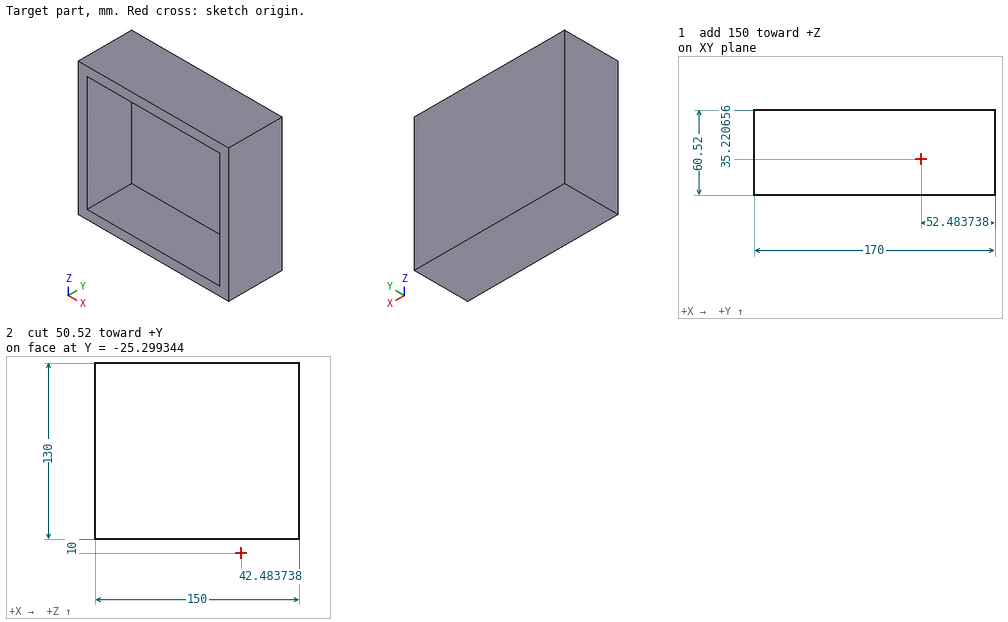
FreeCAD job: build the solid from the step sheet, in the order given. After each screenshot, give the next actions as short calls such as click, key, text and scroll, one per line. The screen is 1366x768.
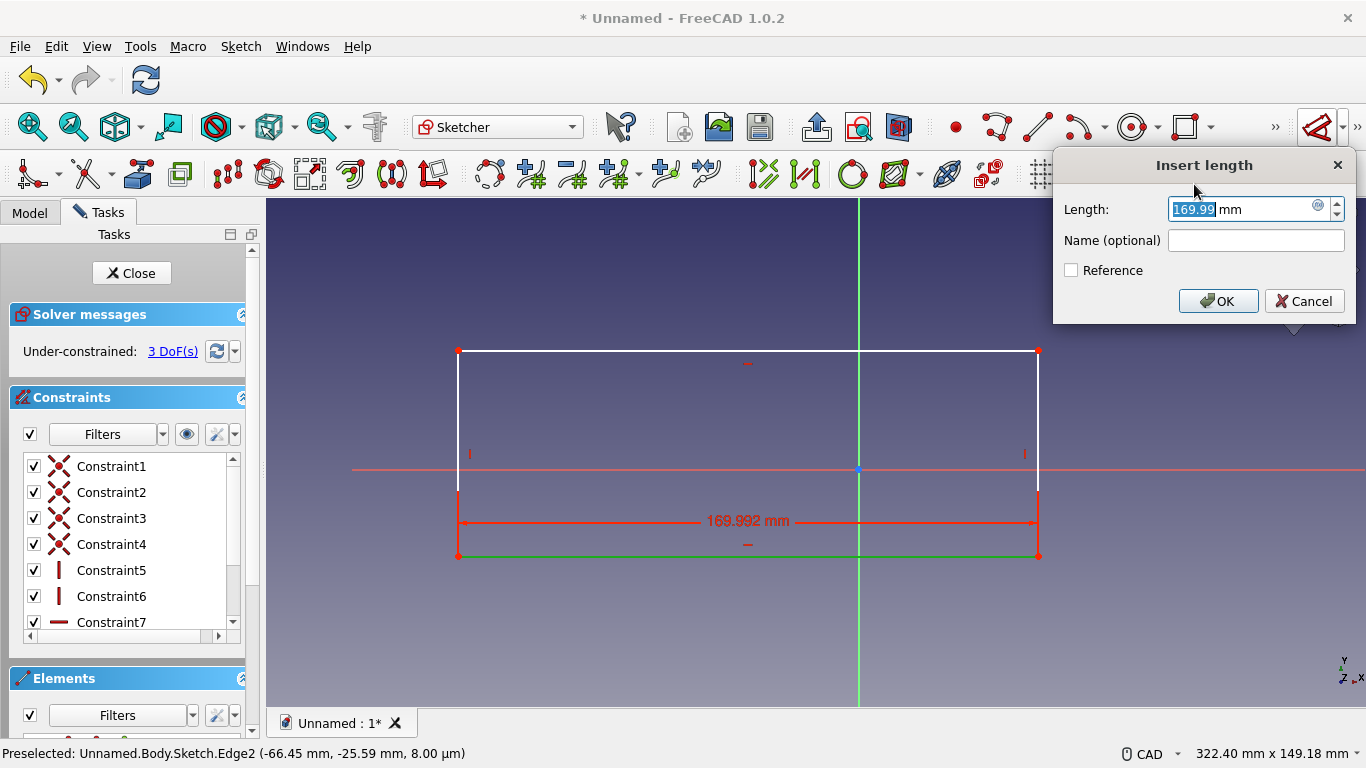
text(170)
key(Return)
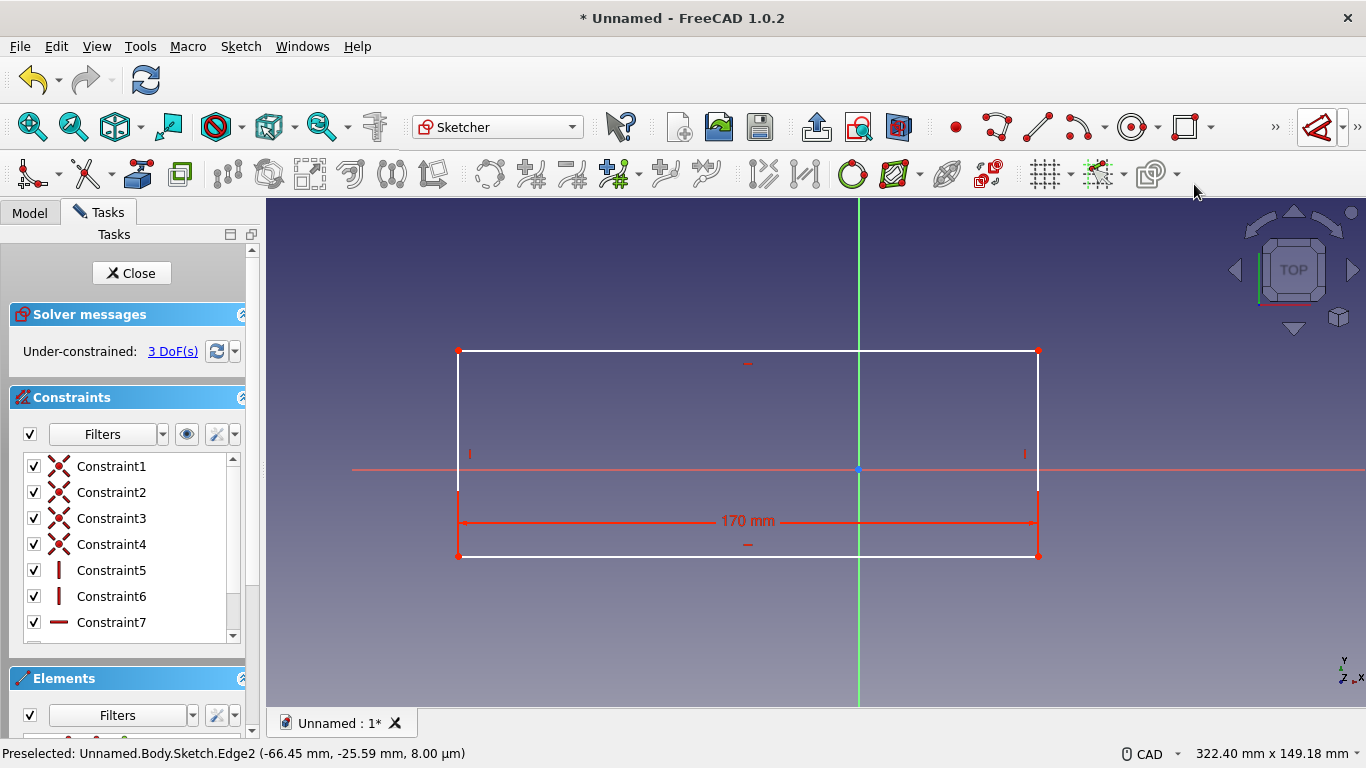
click(458, 413)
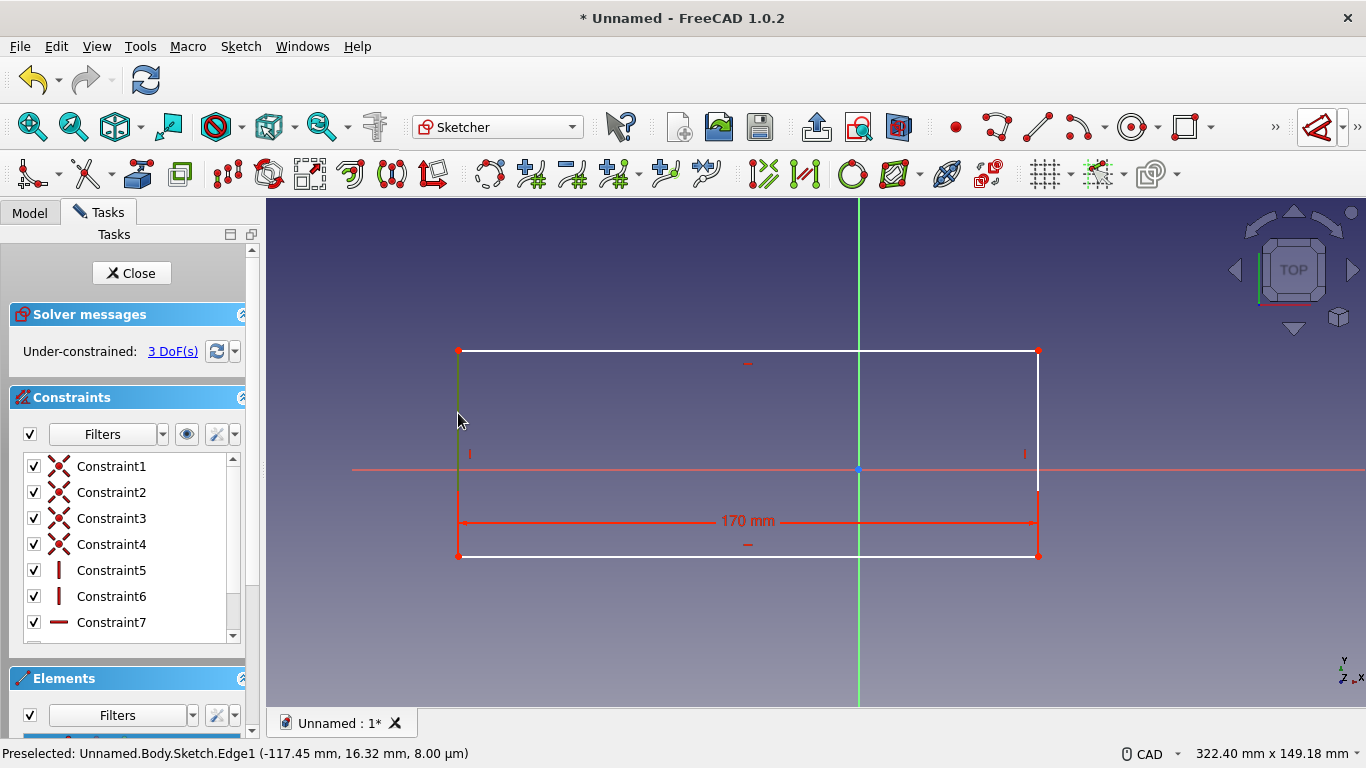
key(i)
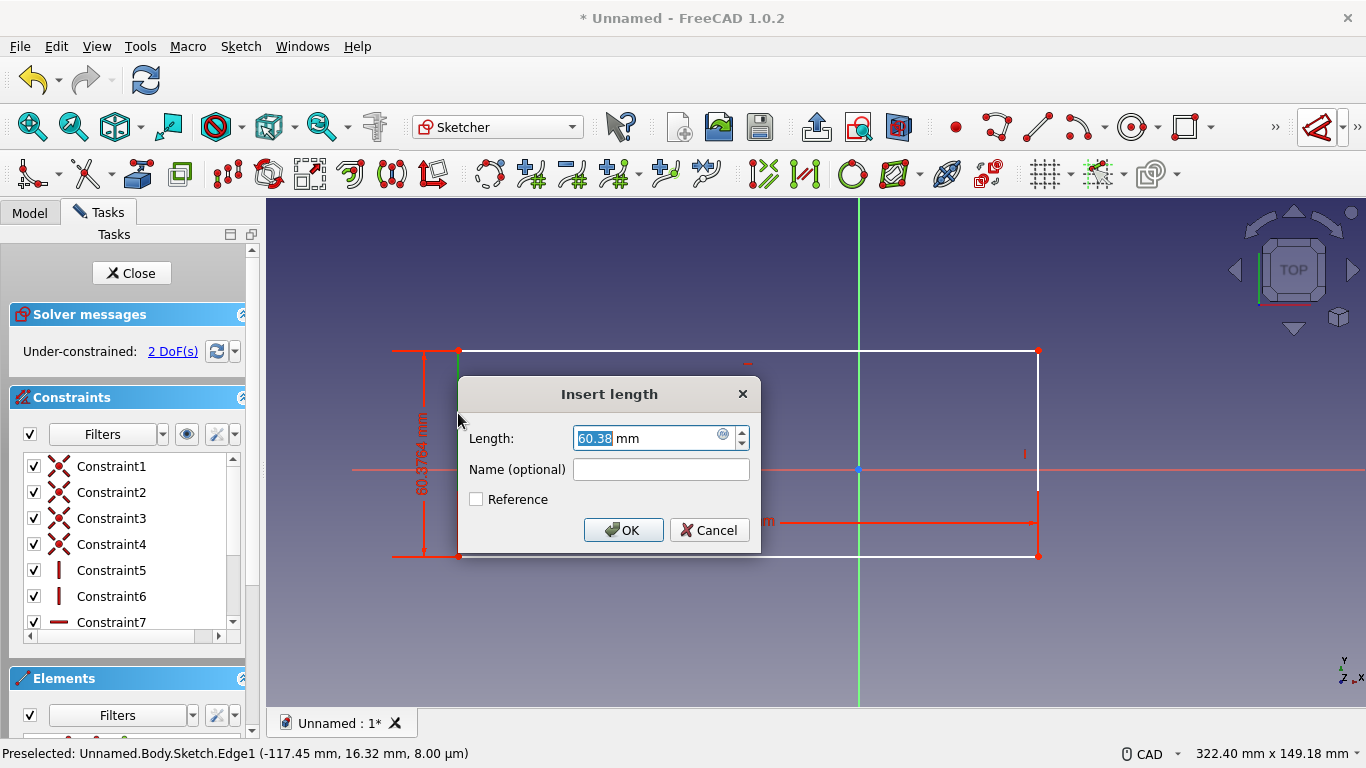
text(60.52)
key(Return)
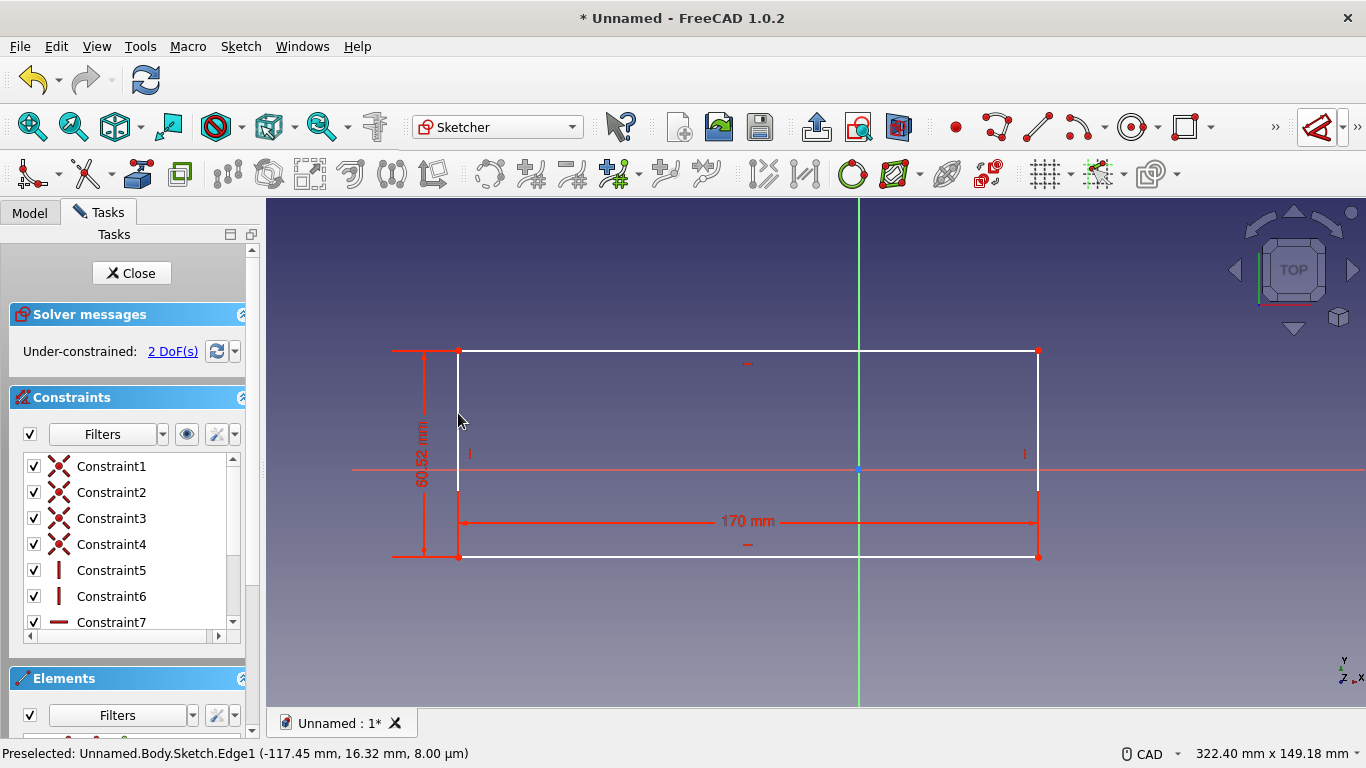
click(458, 351)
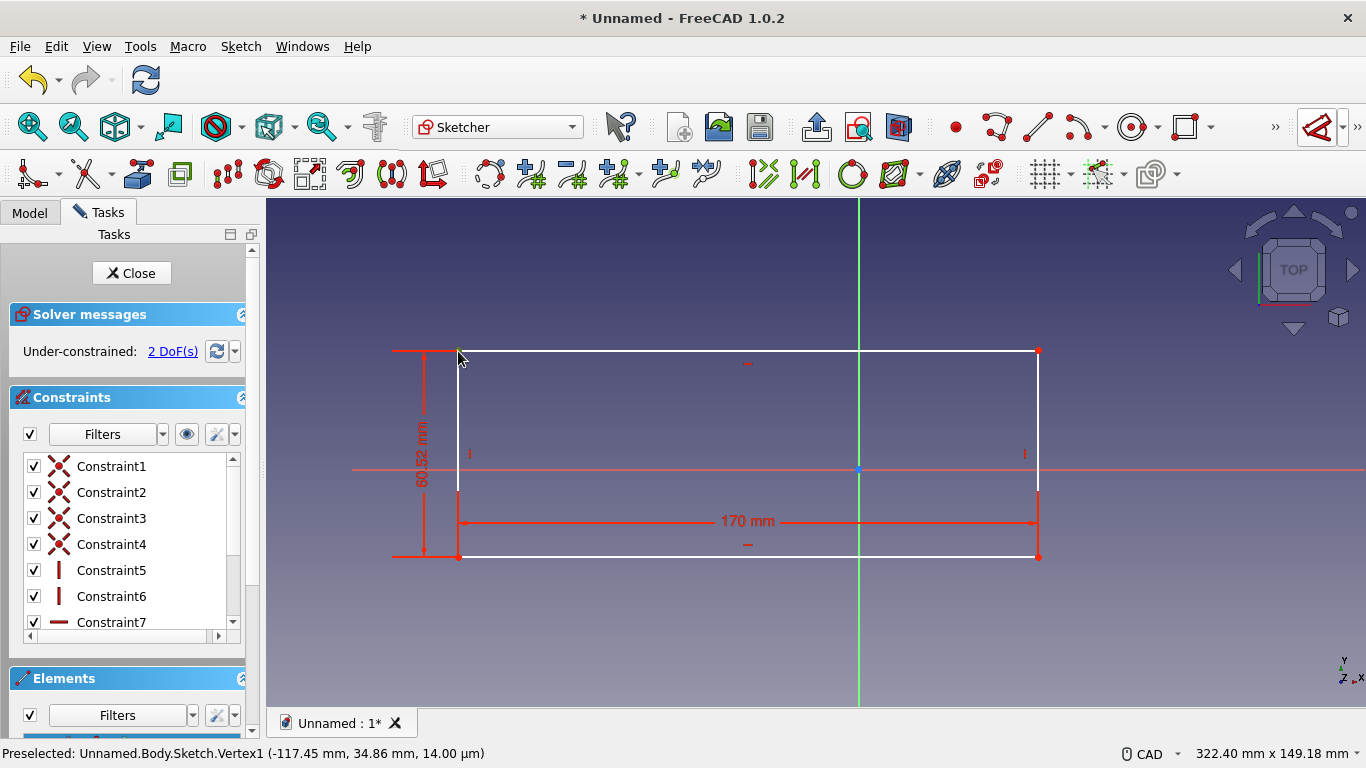
key(i)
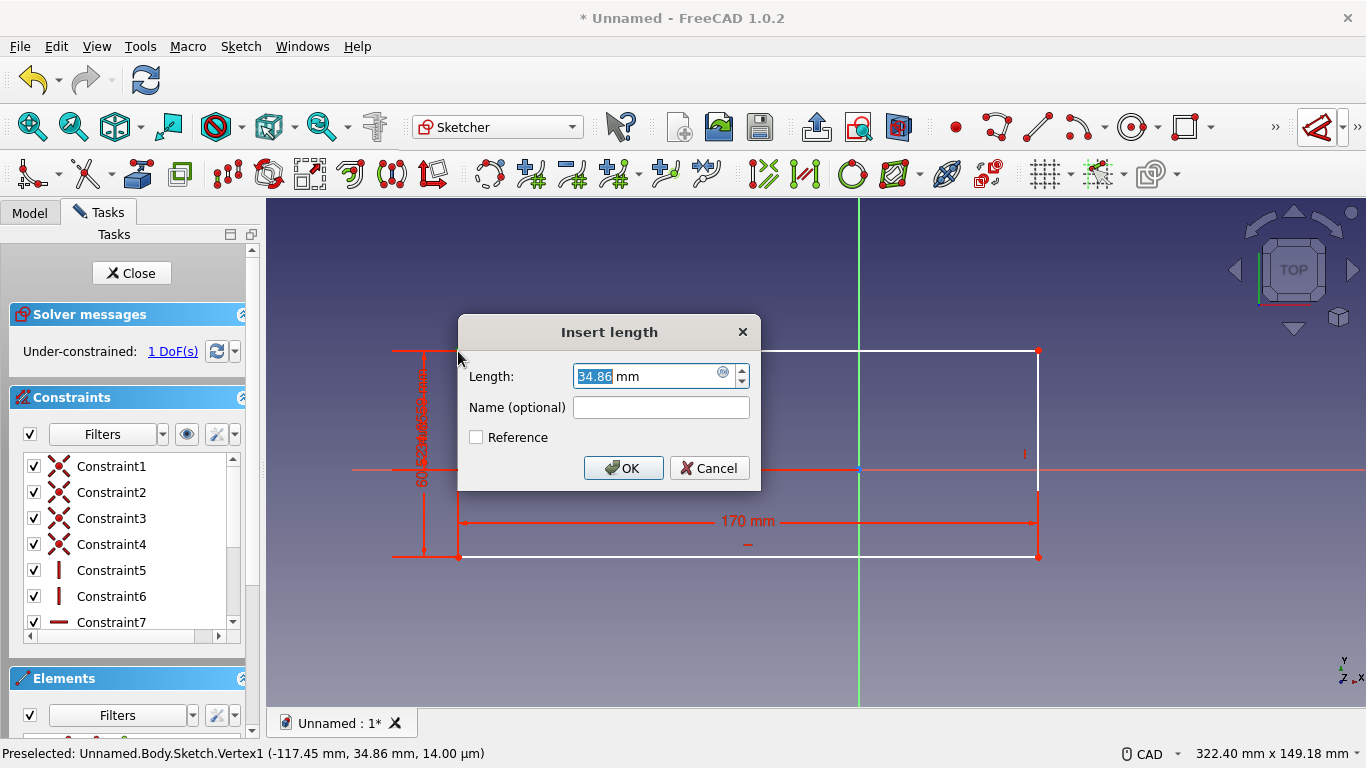
text(35.220656)
key(Return)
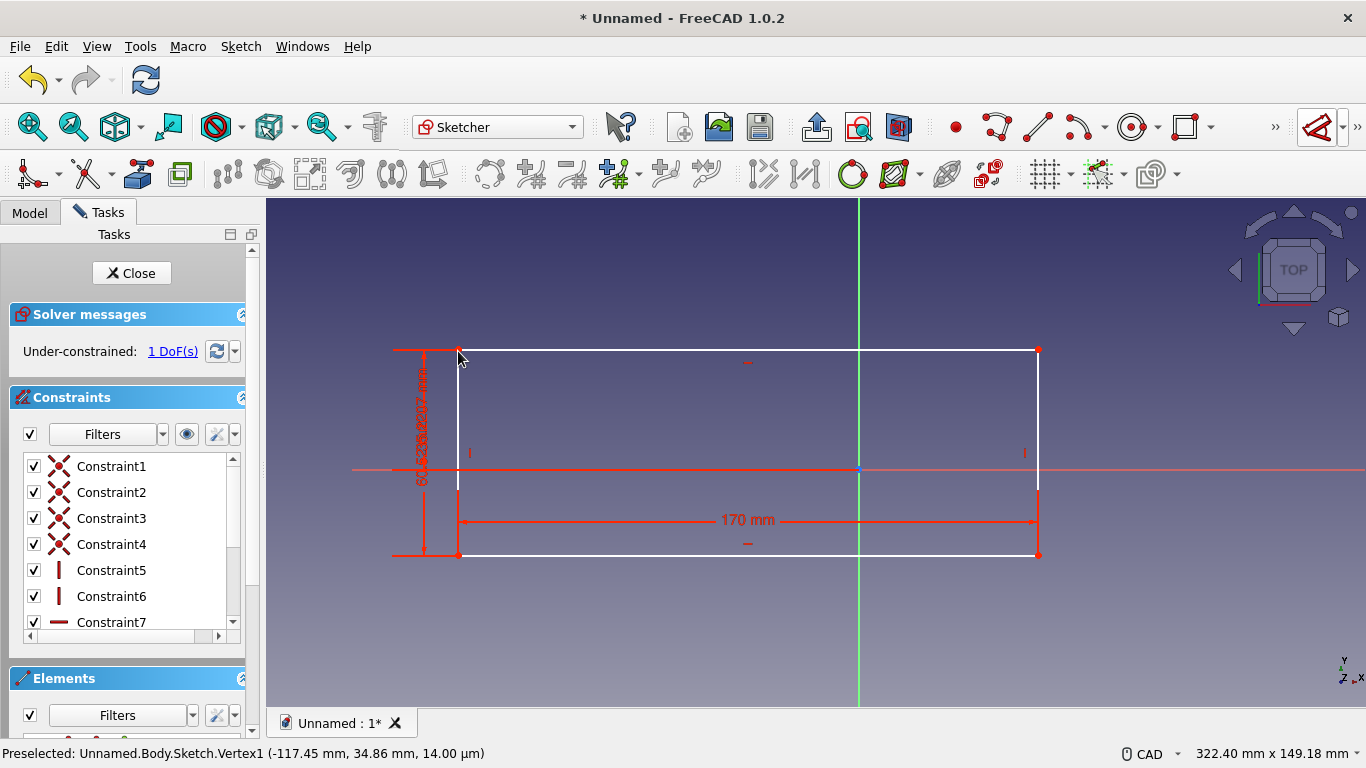
click(1038, 556)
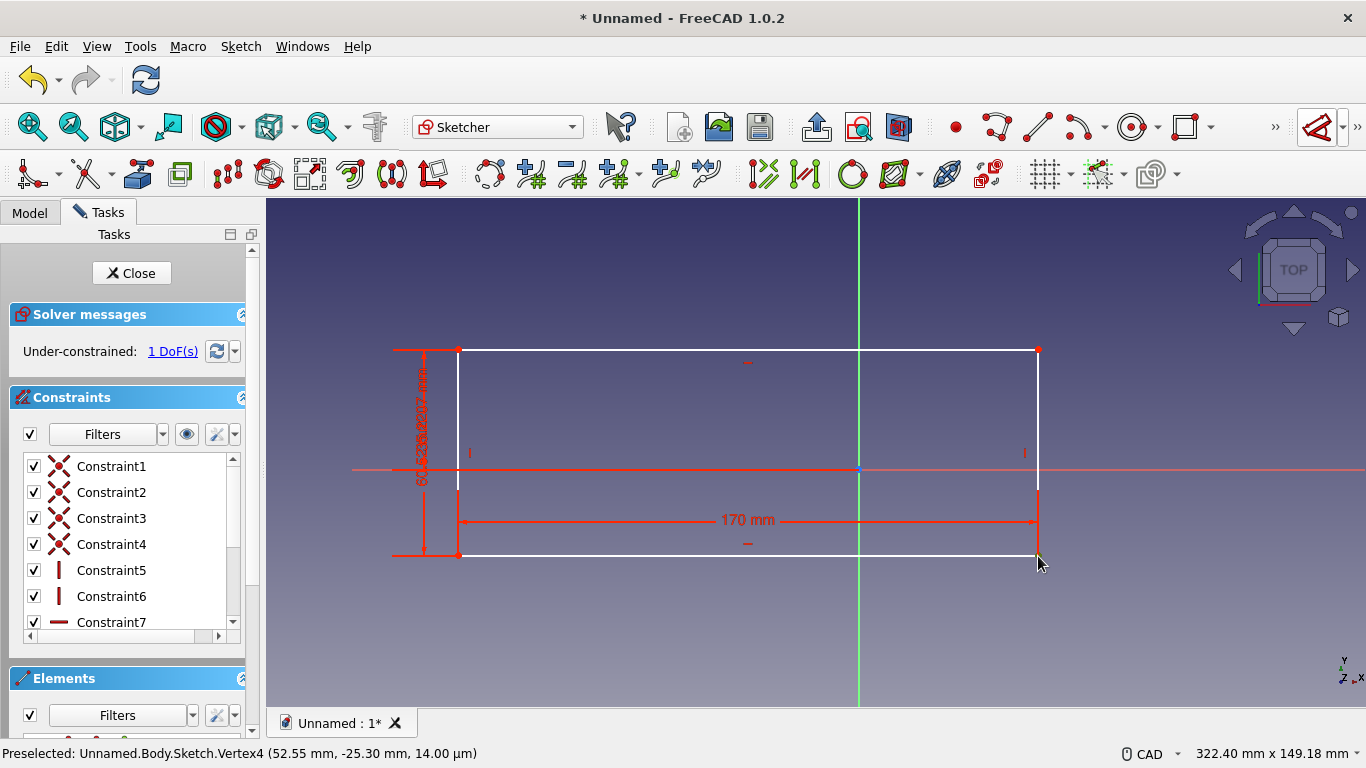
click(1342, 128)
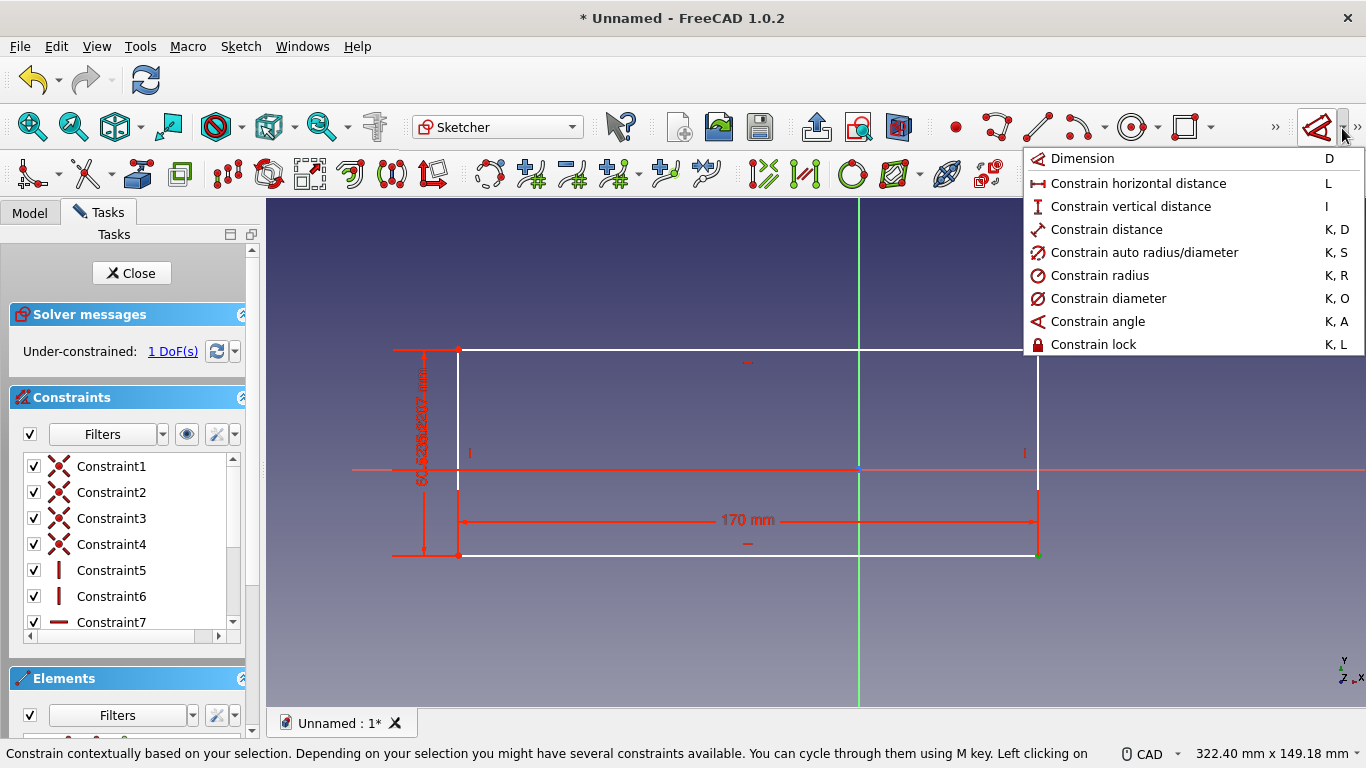
click(1194, 184)